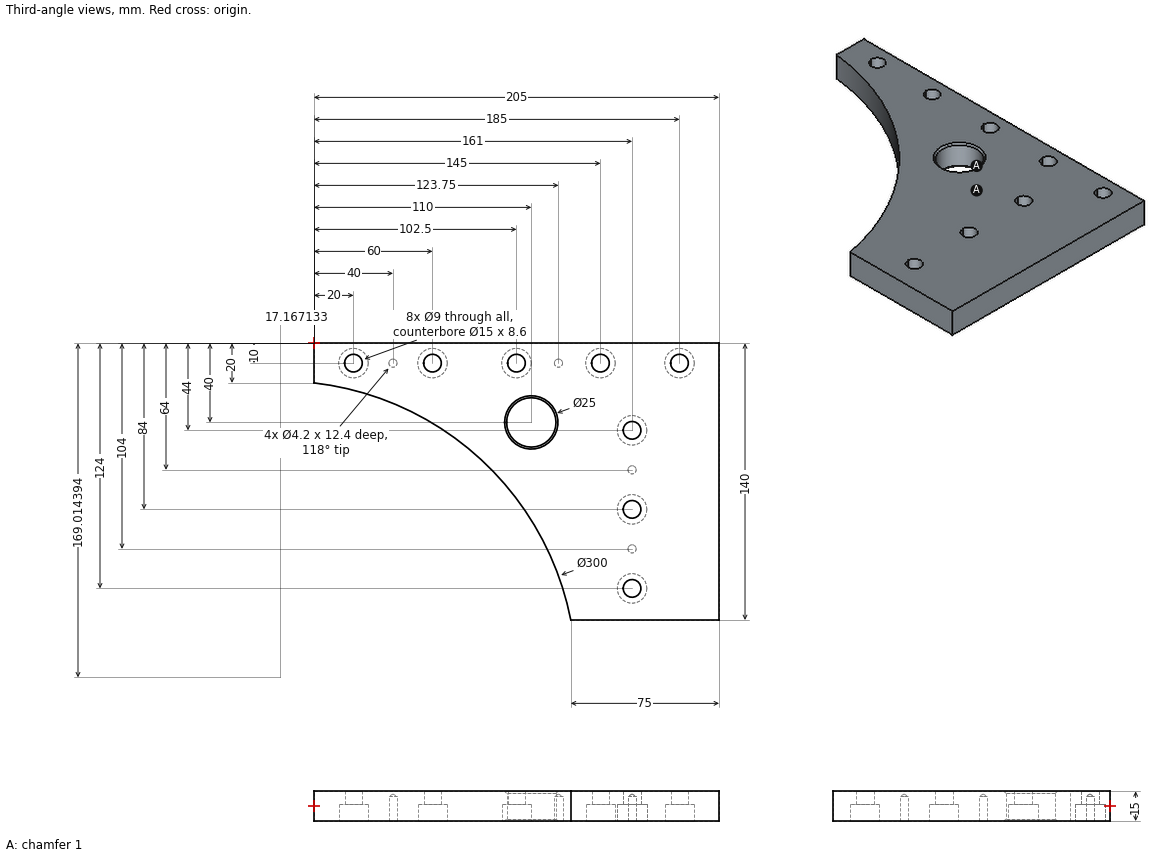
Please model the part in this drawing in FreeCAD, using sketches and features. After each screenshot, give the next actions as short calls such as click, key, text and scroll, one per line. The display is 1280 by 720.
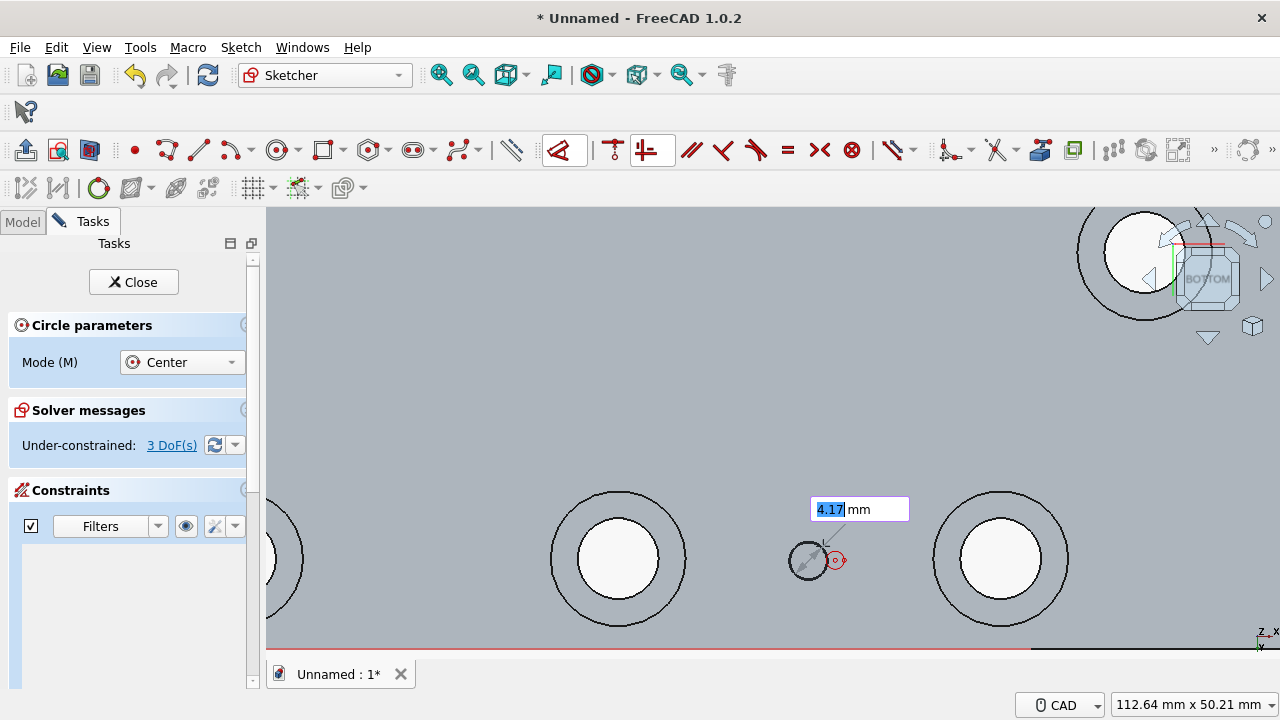
click(823, 545)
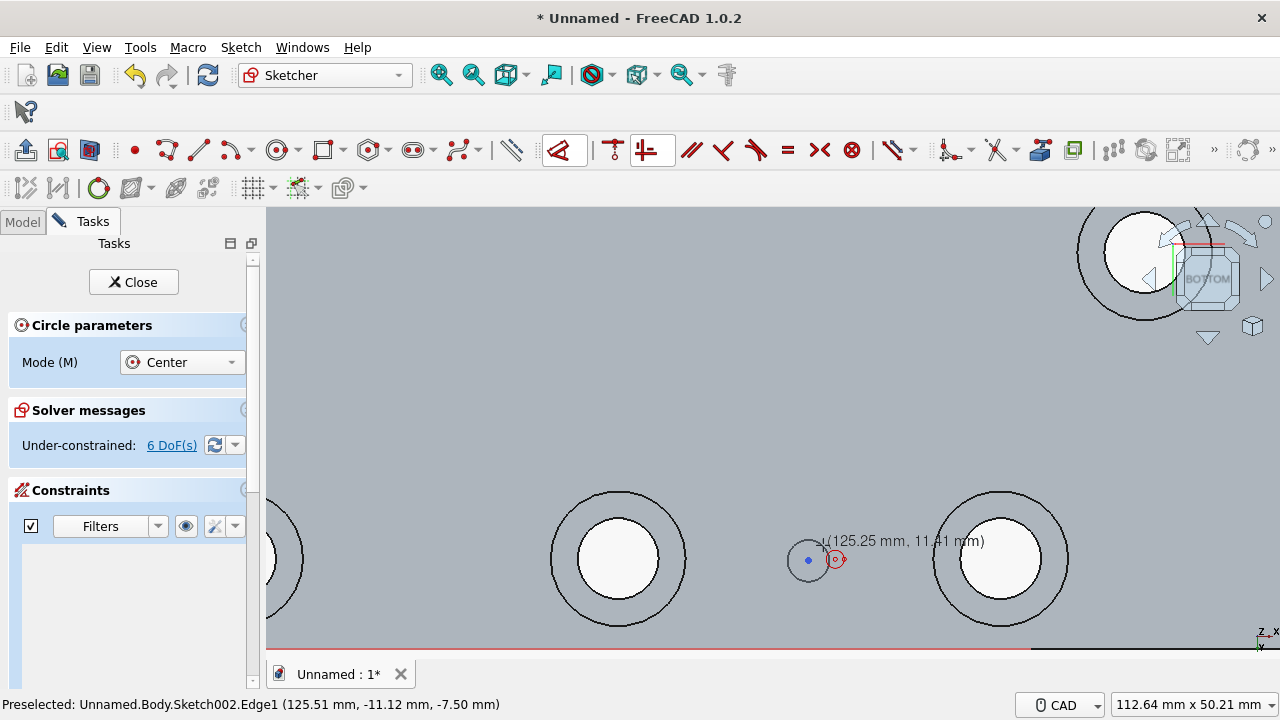
scroll(823, 546, down, 6)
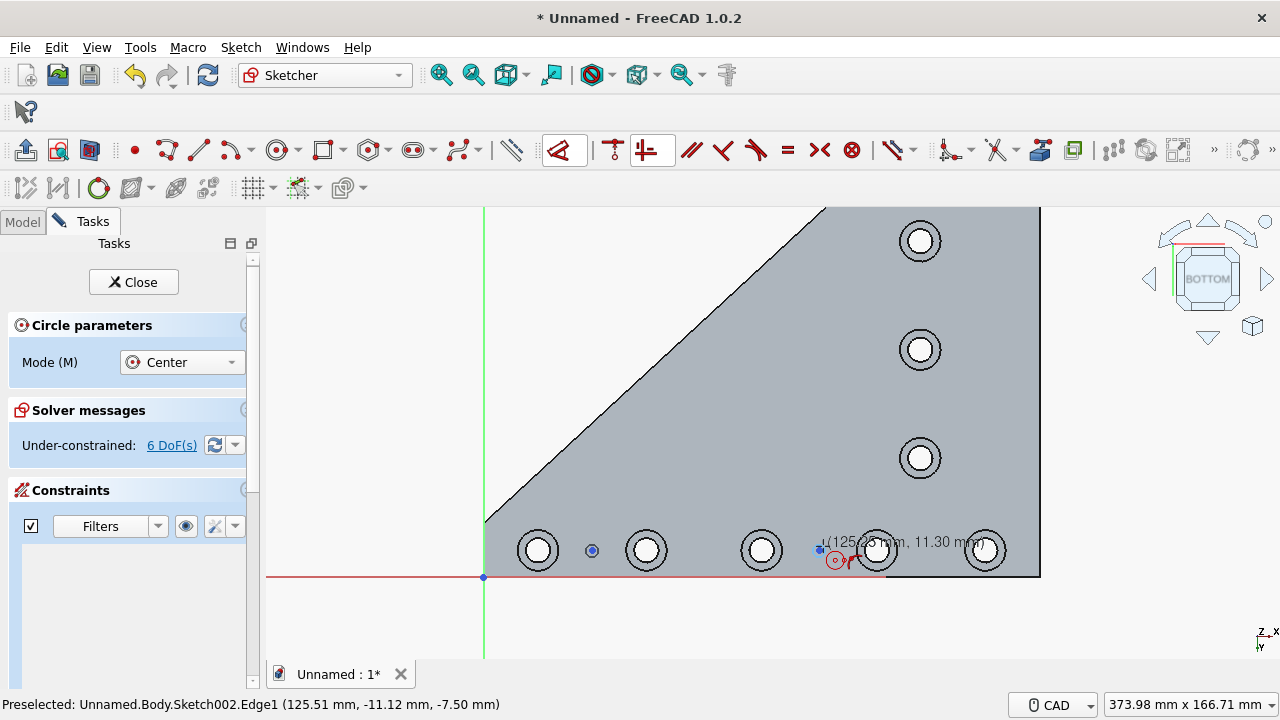
scroll(920, 404, up, 7)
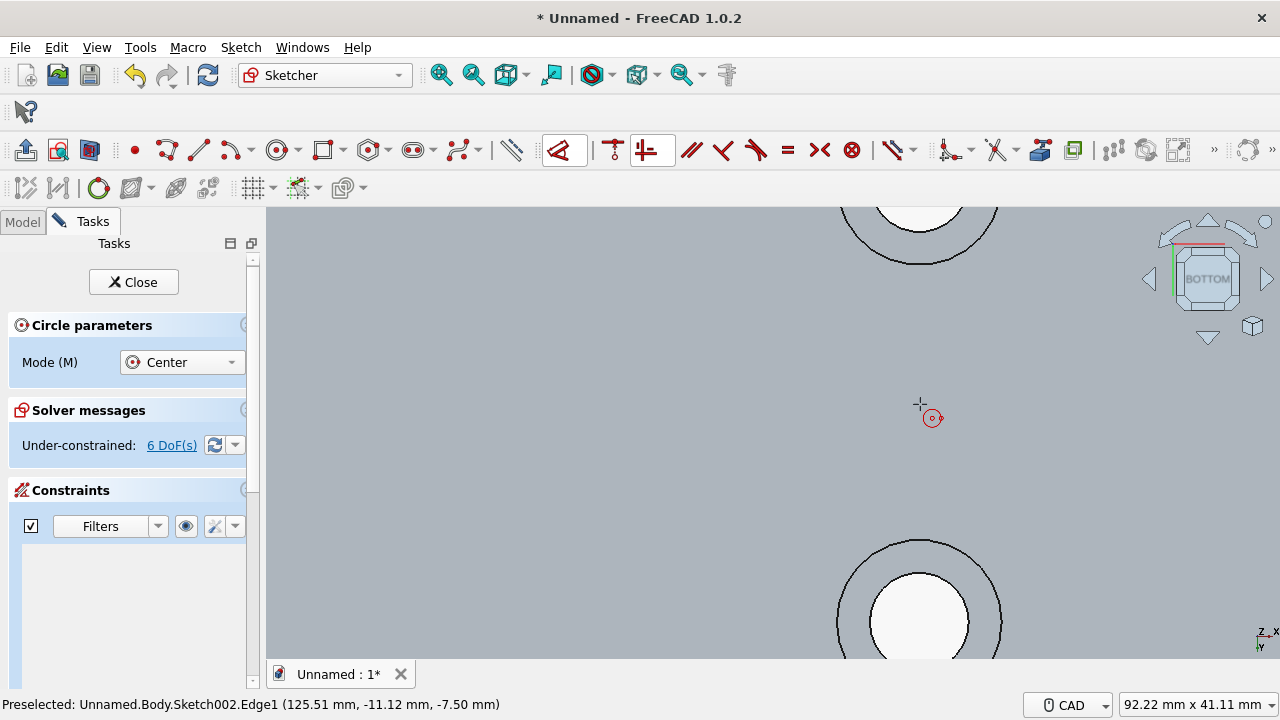
scroll(920, 404, down, 7)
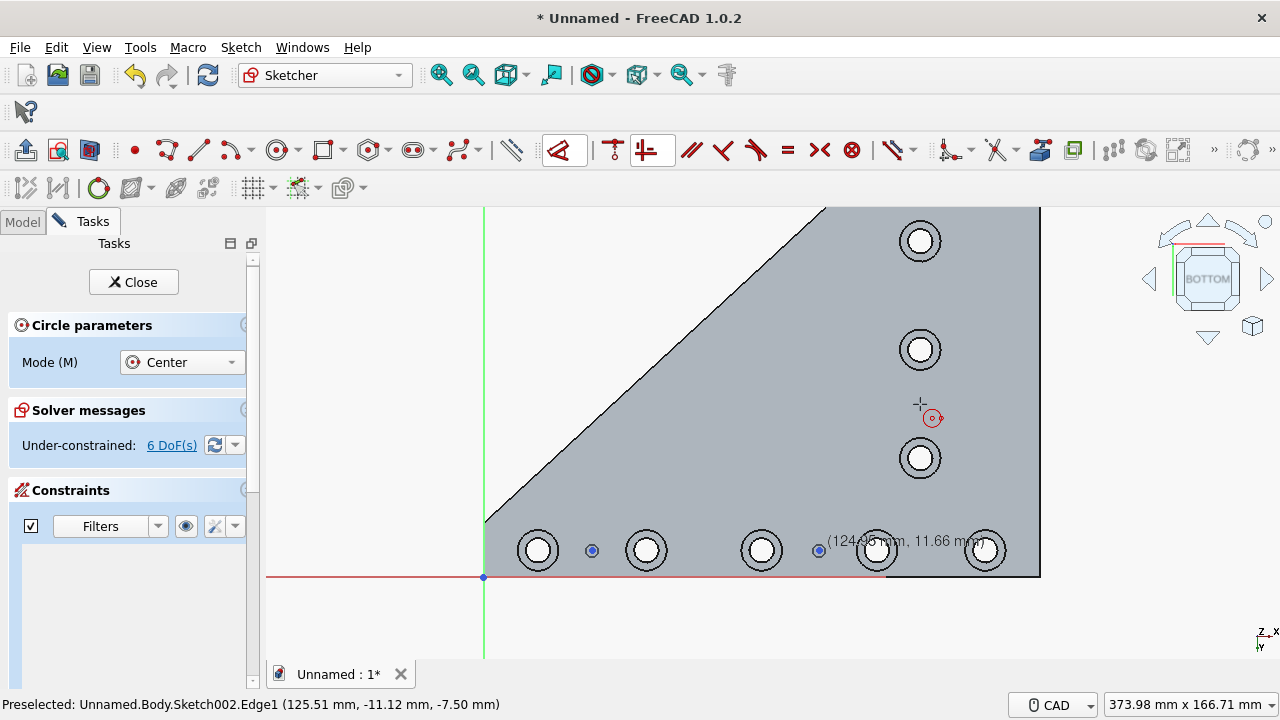
click(920, 404)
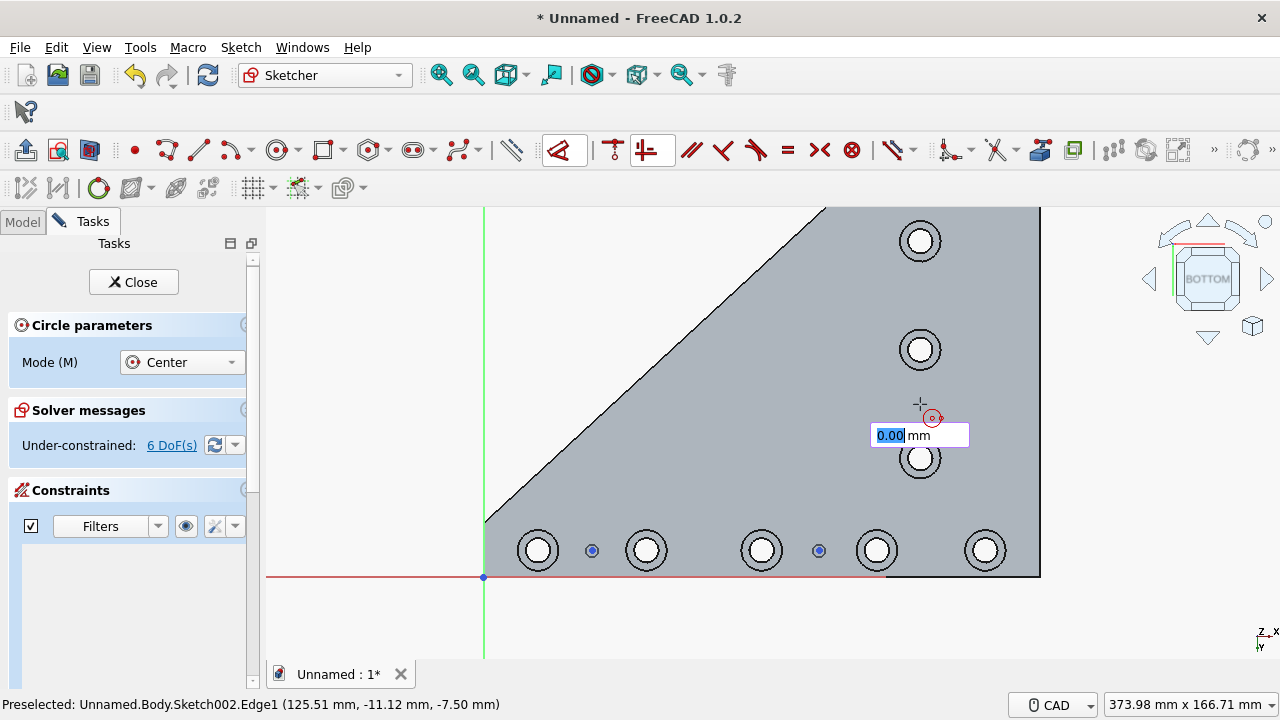
scroll(924, 400, up, 6)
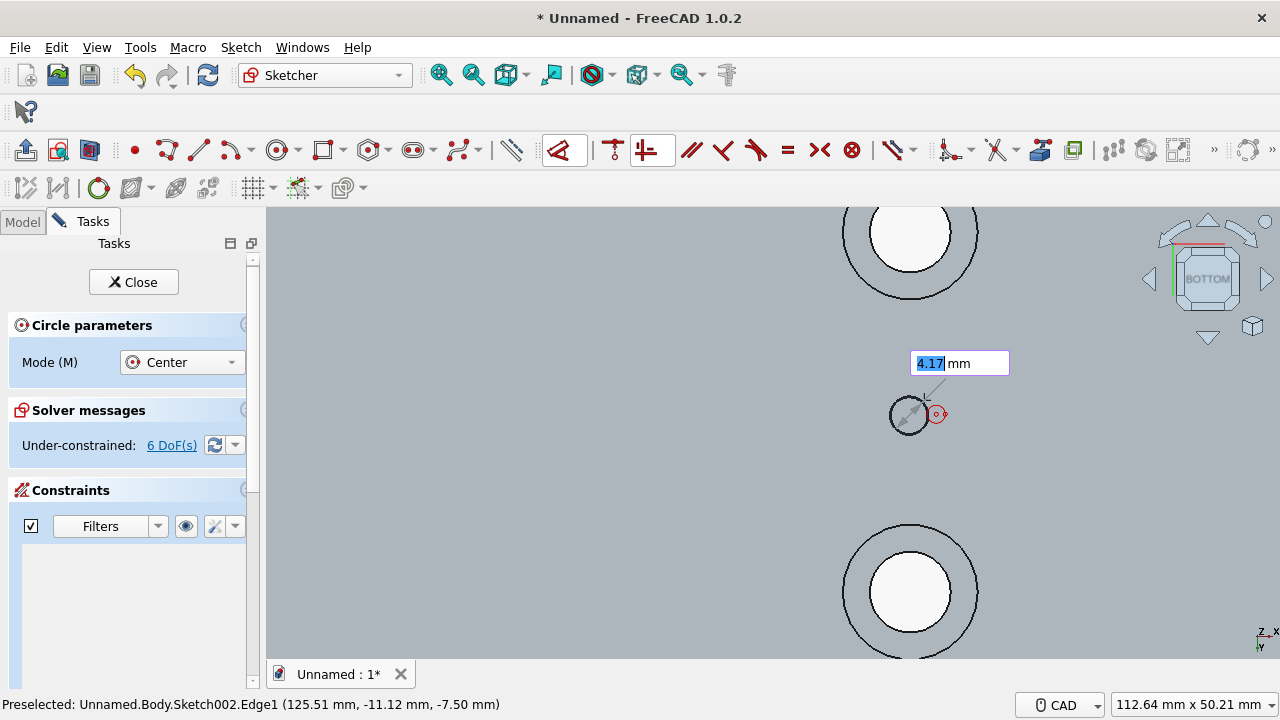
click(924, 399)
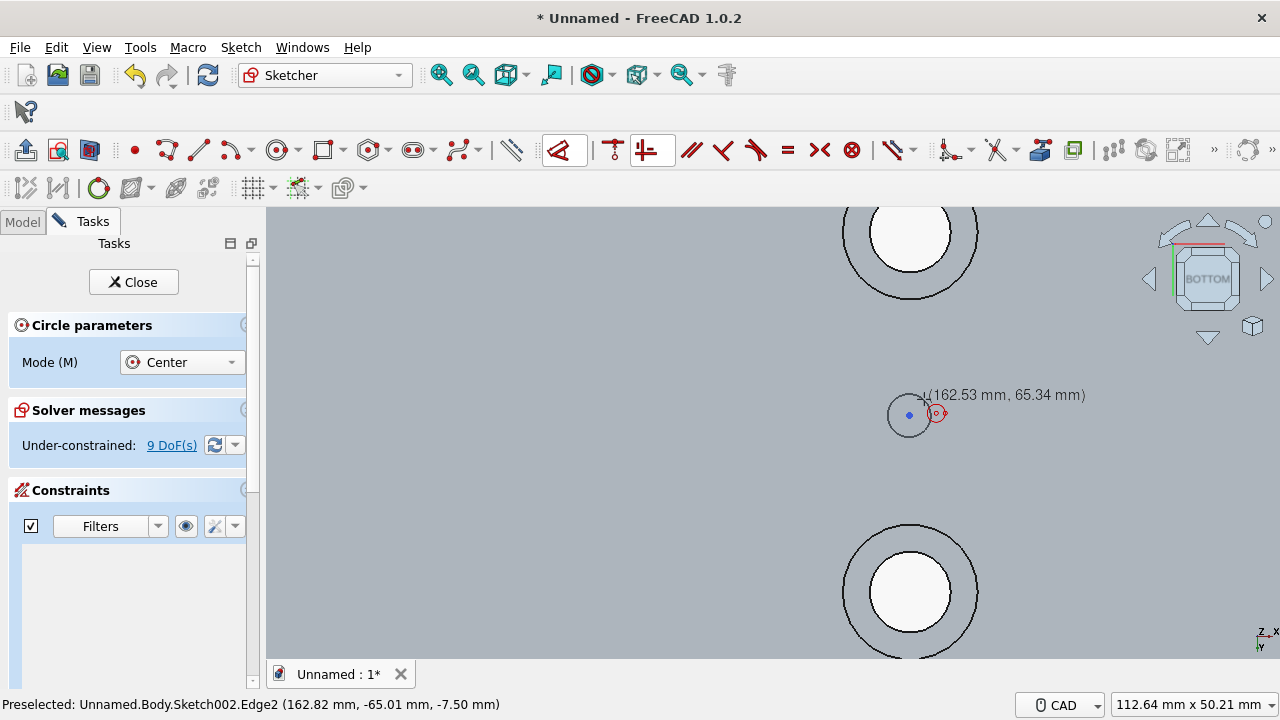
scroll(924, 400, down, 6)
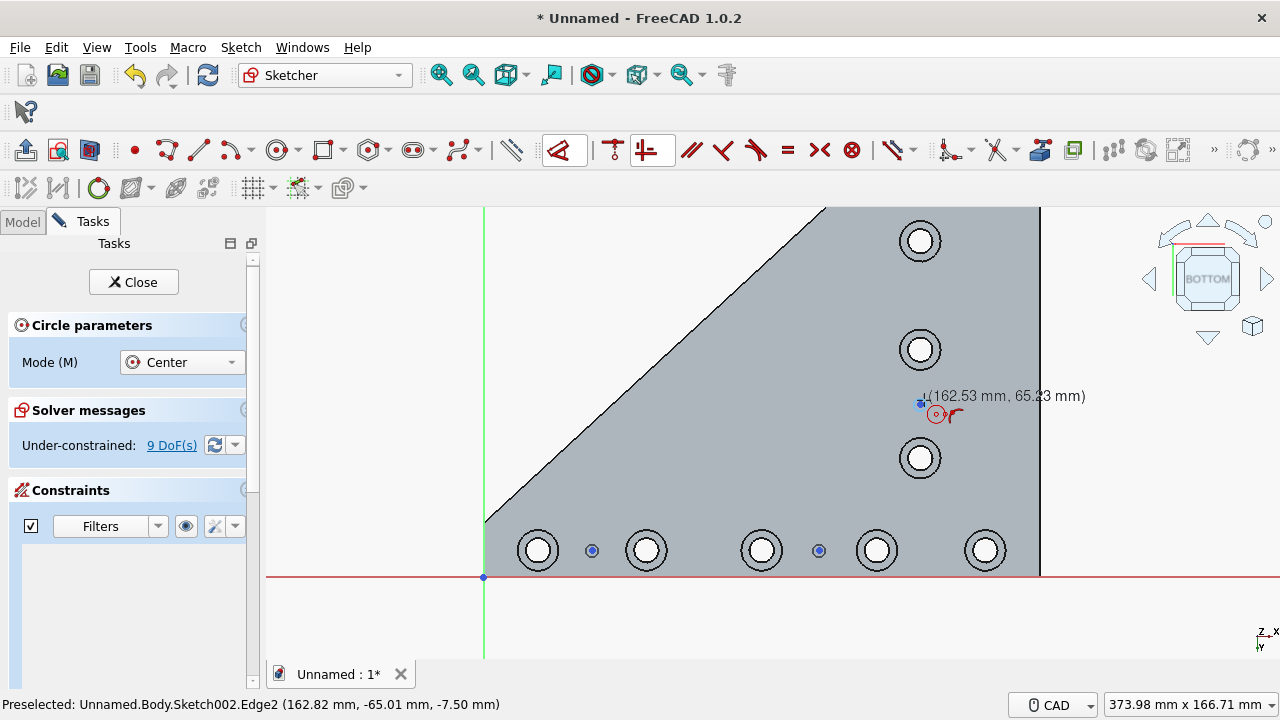
scroll(920, 295, up, 7)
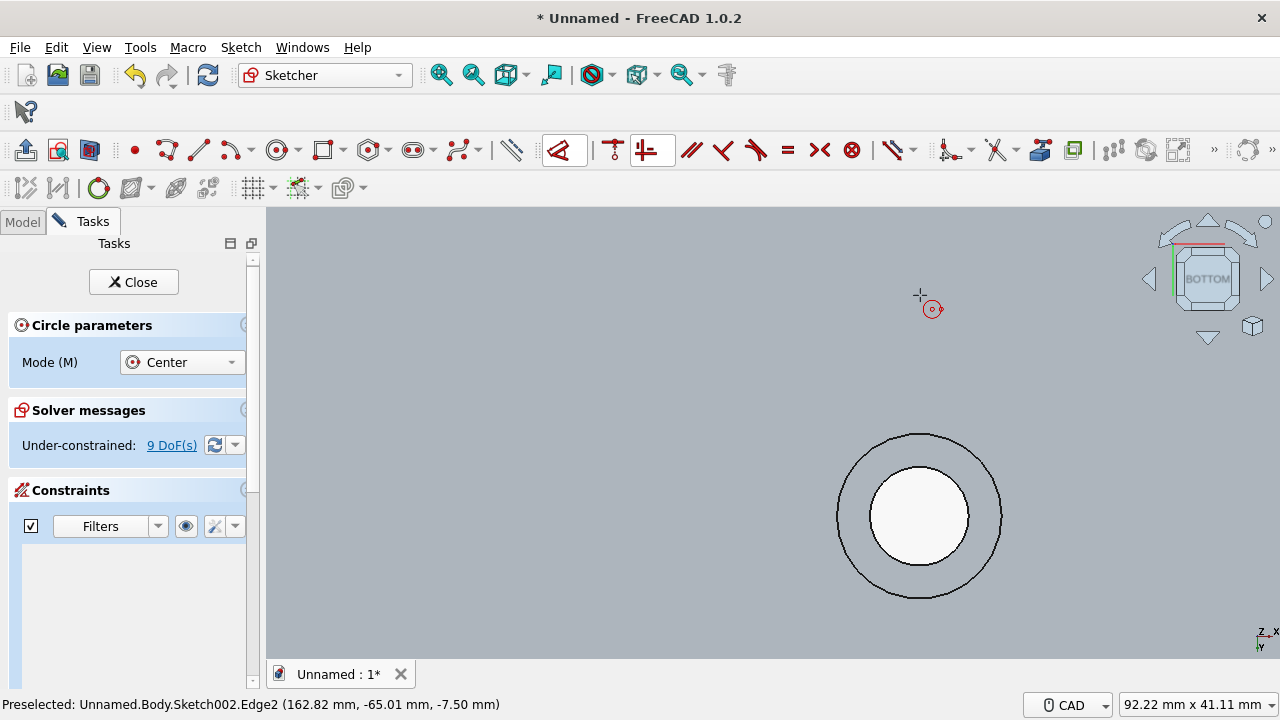
scroll(920, 294, down, 7)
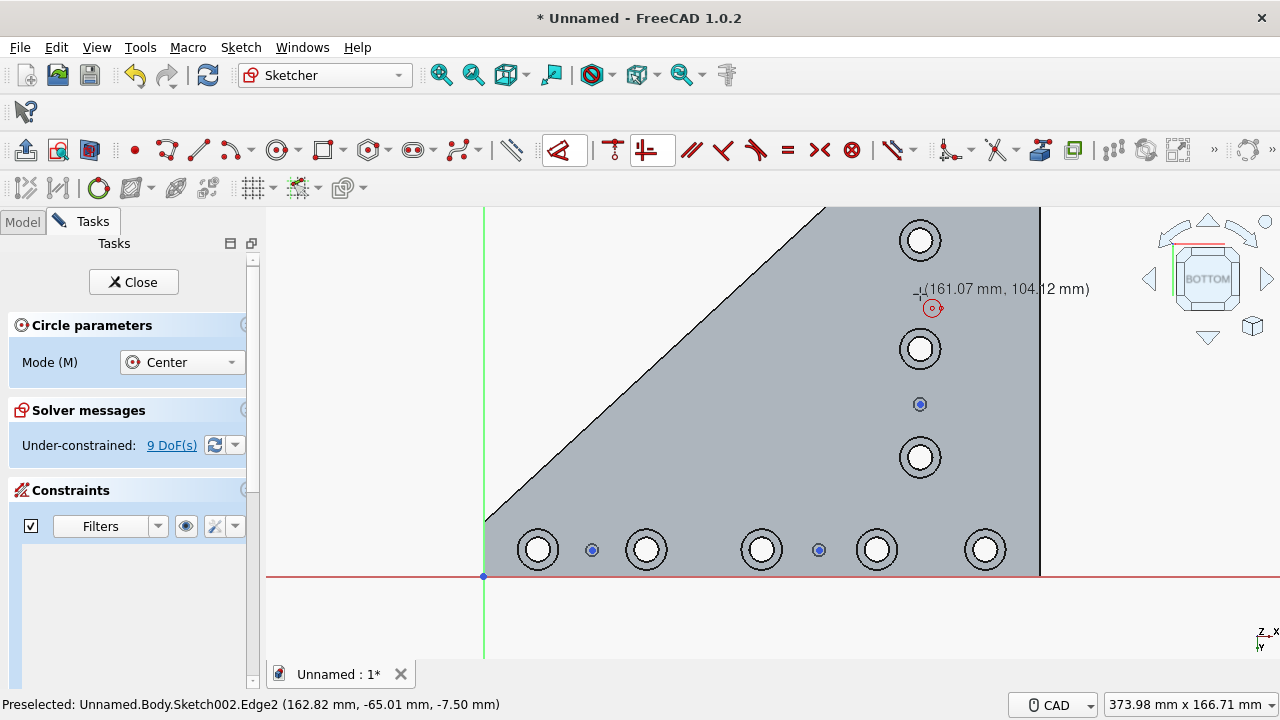
click(920, 295)